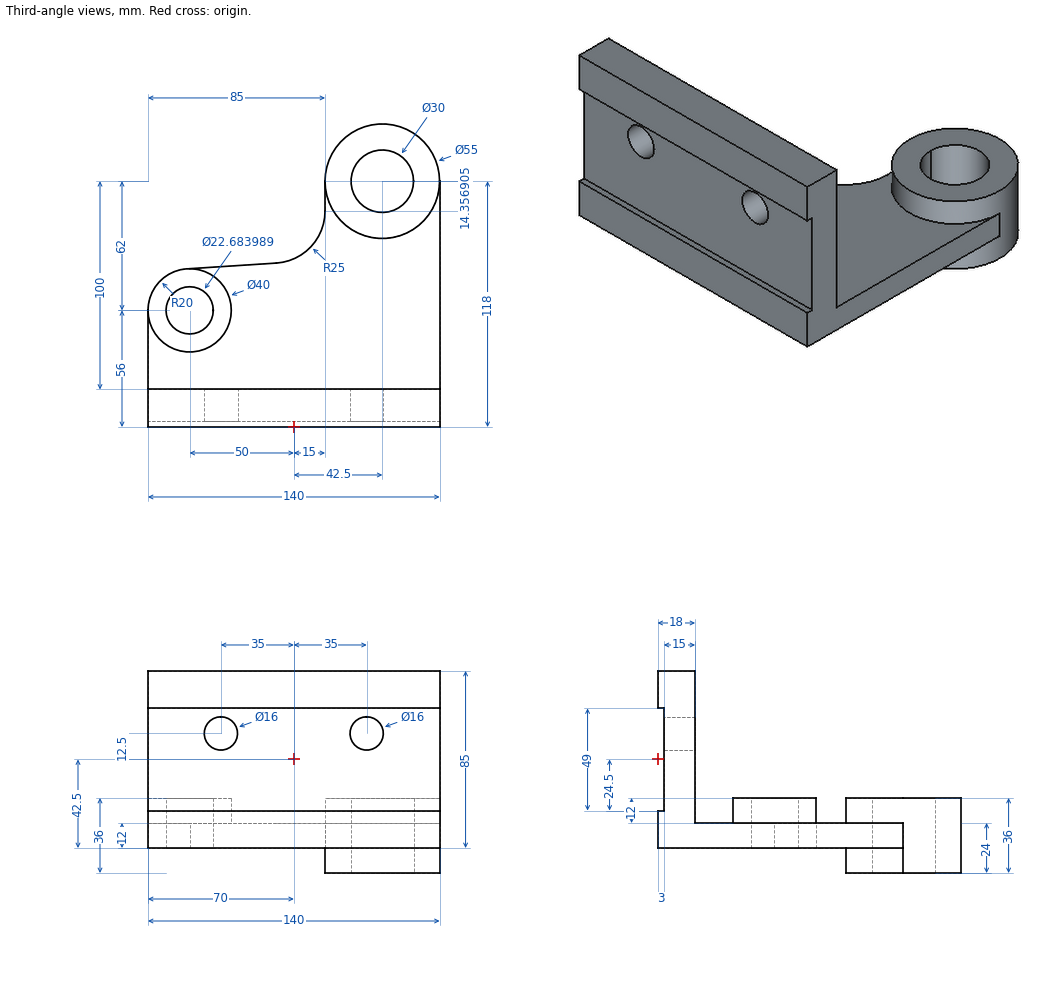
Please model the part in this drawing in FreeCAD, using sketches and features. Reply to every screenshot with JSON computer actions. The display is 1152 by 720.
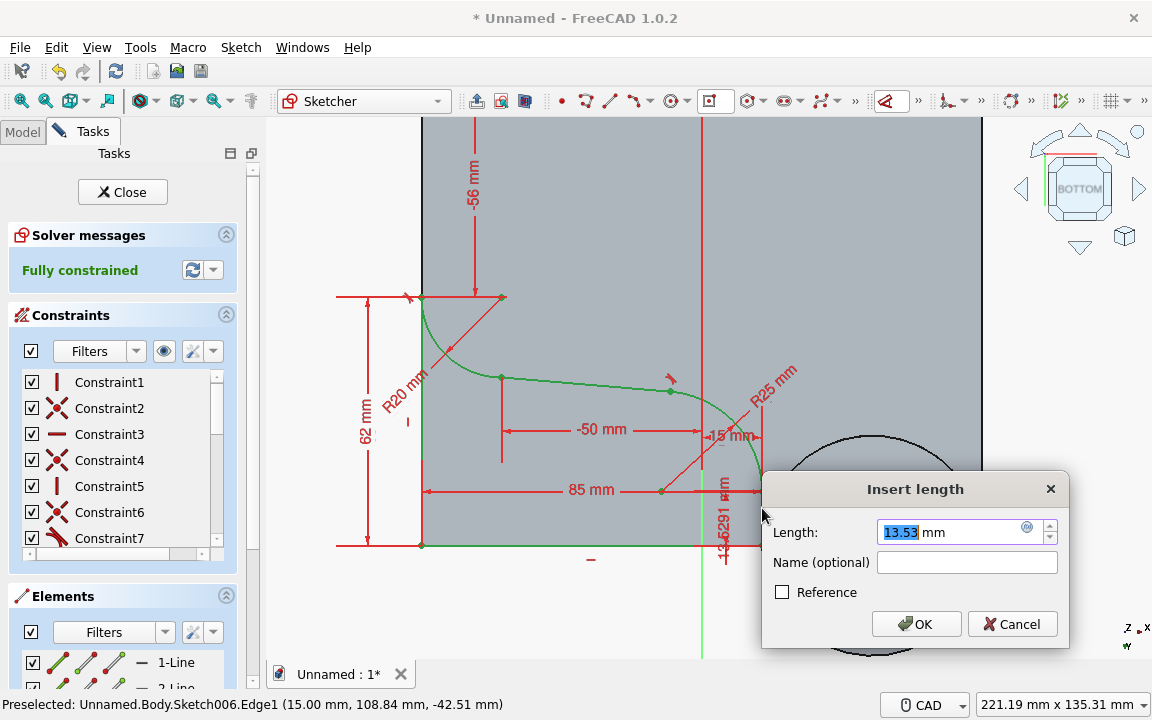
{"action": "type", "text": "14.356905"}
{"action": "key", "text": "Return"}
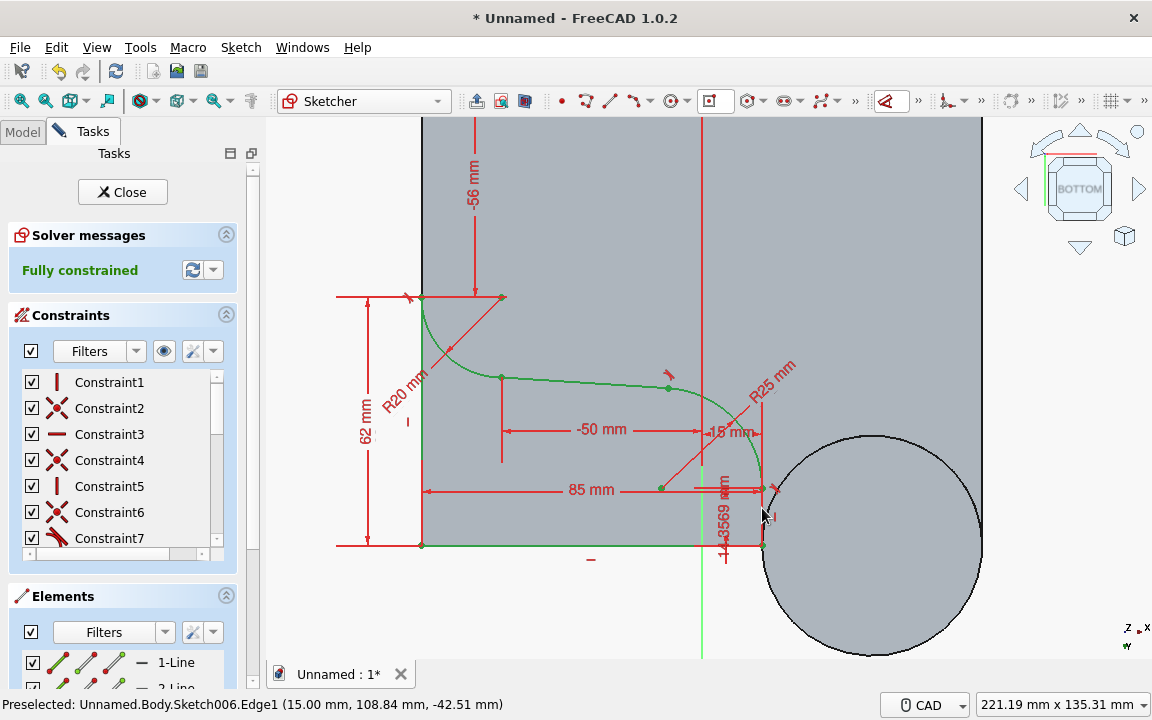
{"action": "left_click", "coordinate": [123, 192]}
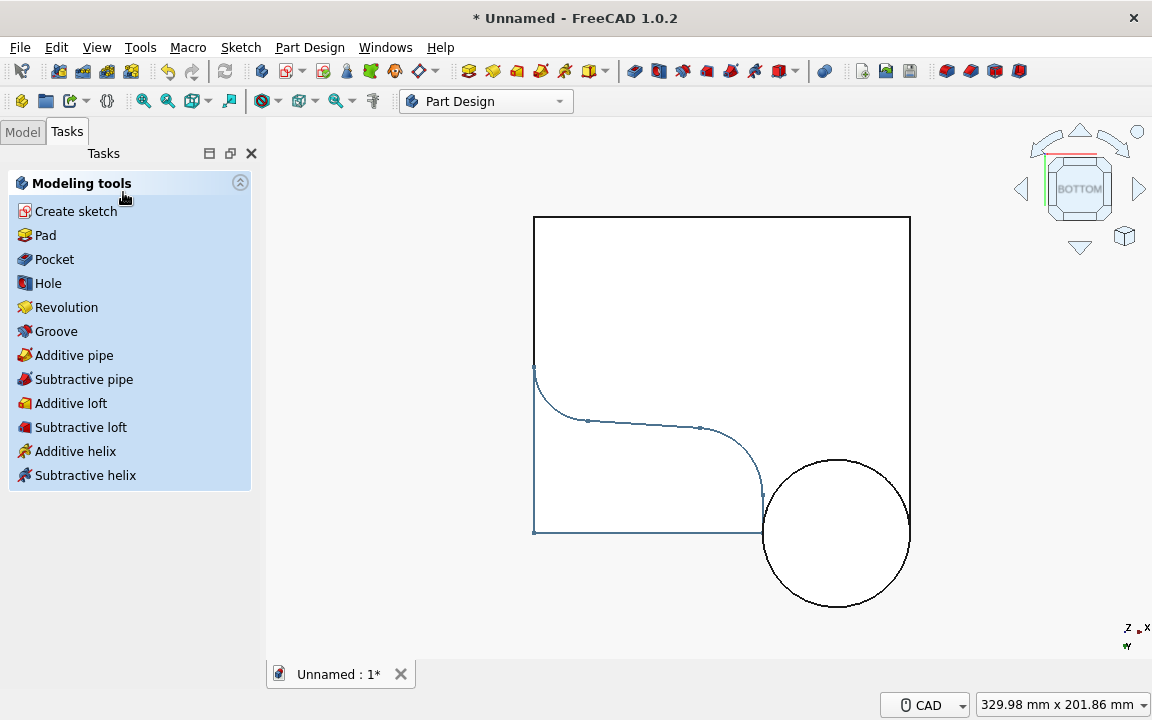
{"action": "left_click", "coordinate": [636, 72]}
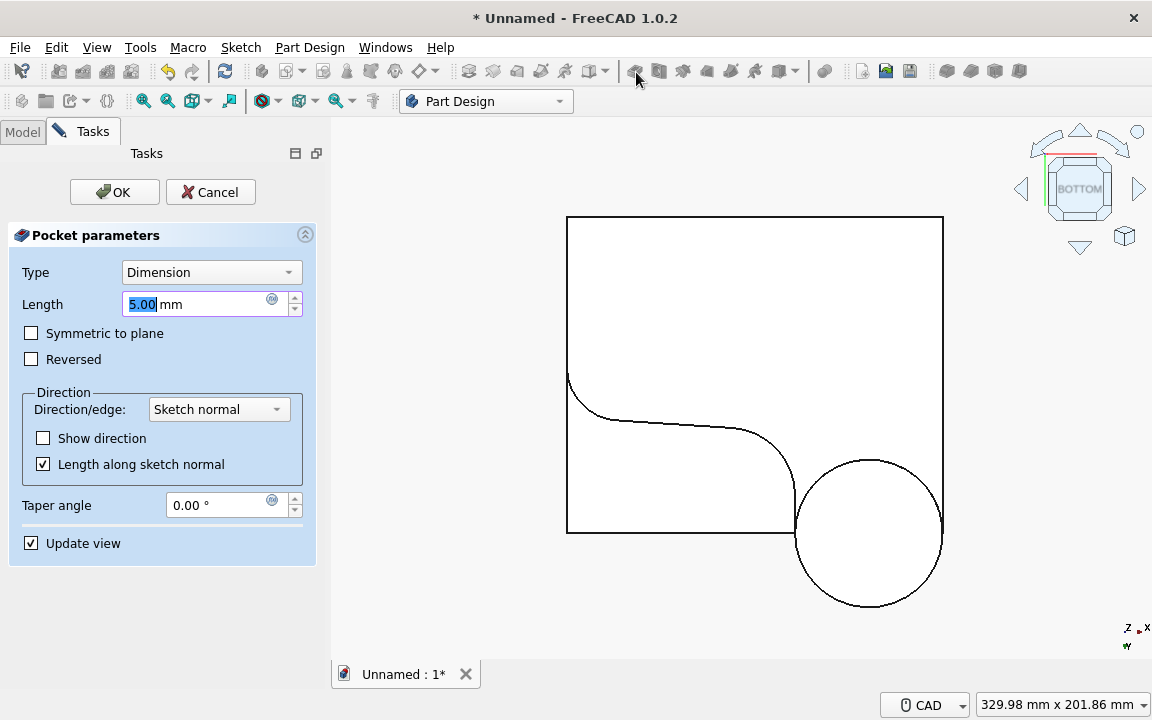
{"action": "type", "text": "12"}
{"action": "key", "text": "Tab"}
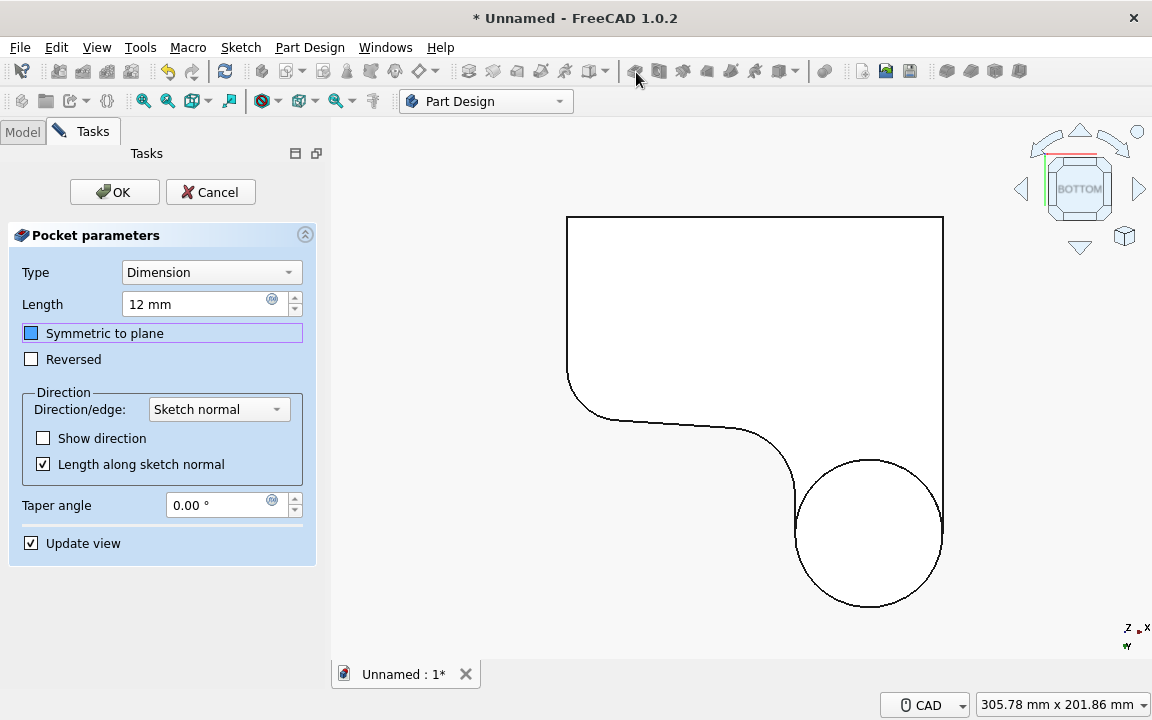
{"action": "left_click", "coordinate": [115, 192]}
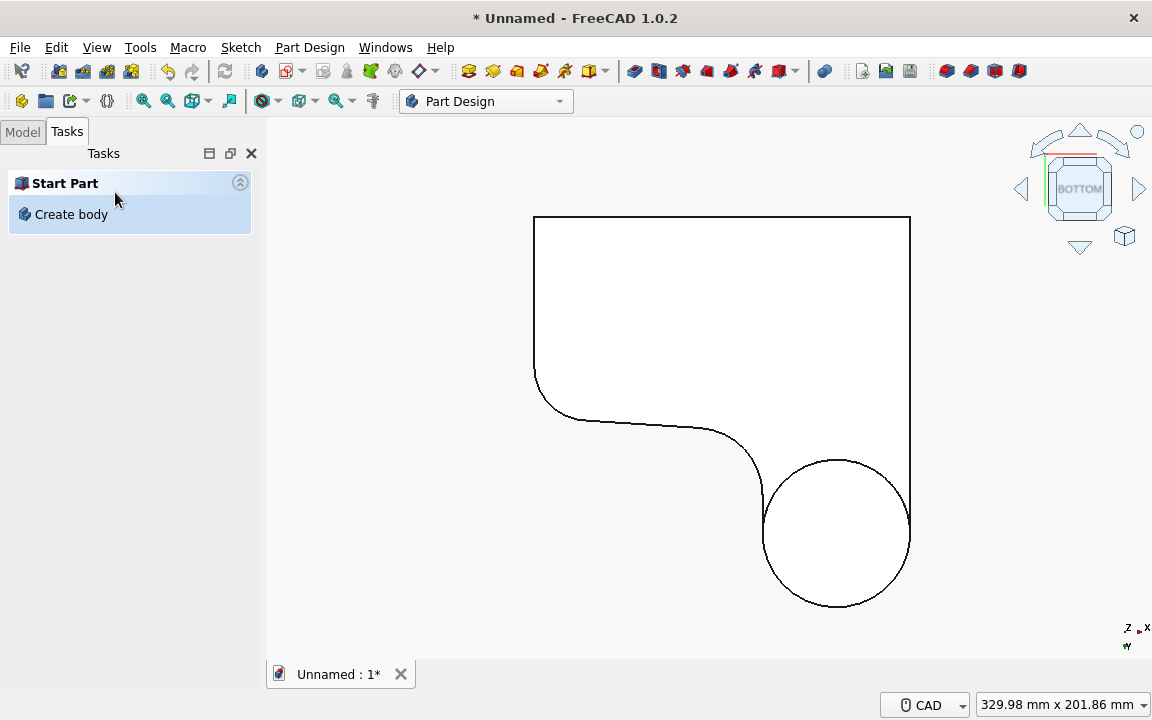
{"action": "key", "text": "0"}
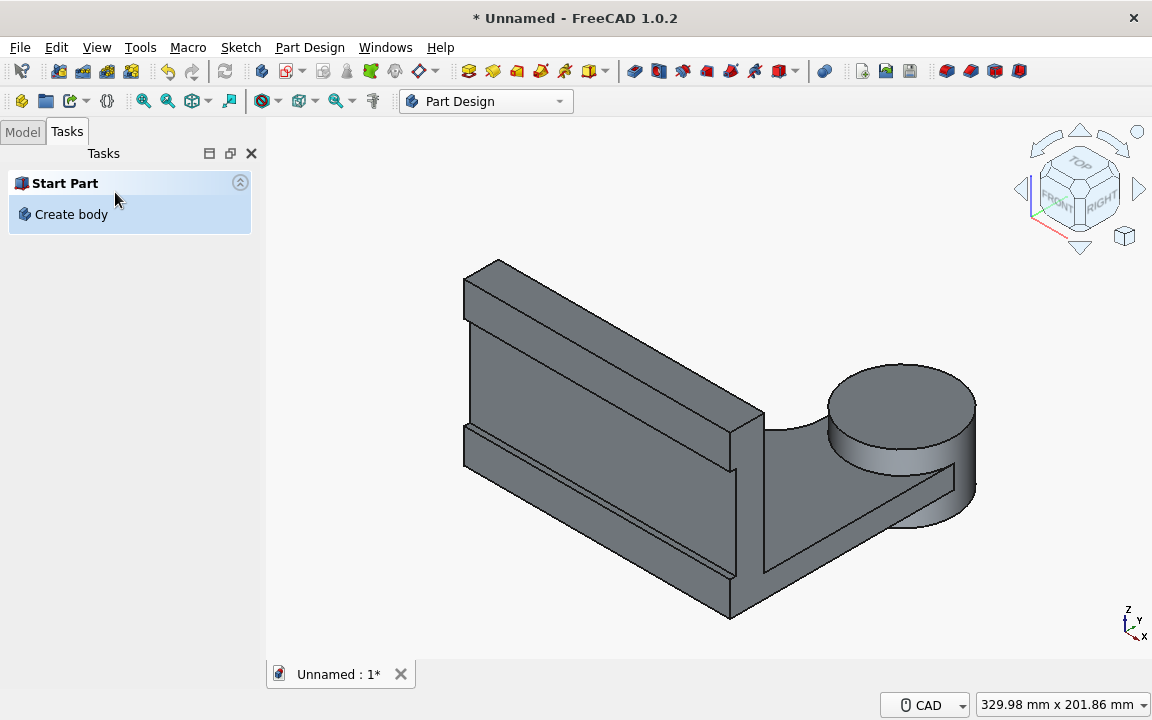
{"action": "left_click", "coordinate": [902, 406]}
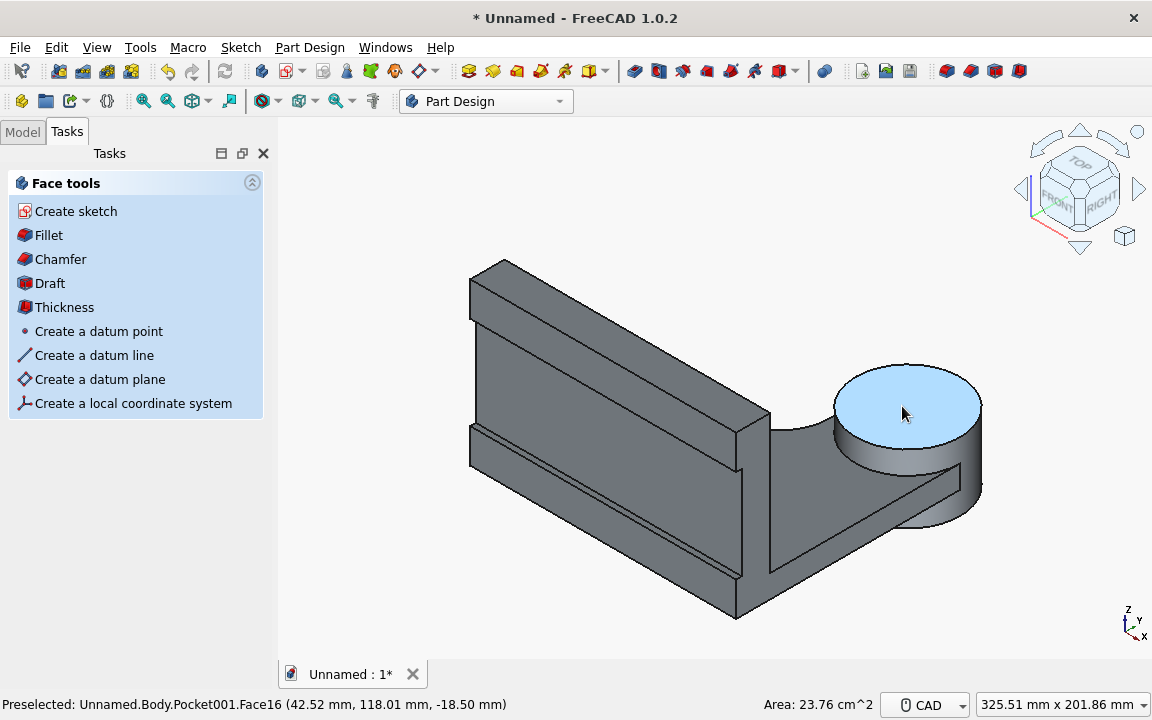
{"action": "left_click", "coordinate": [286, 72]}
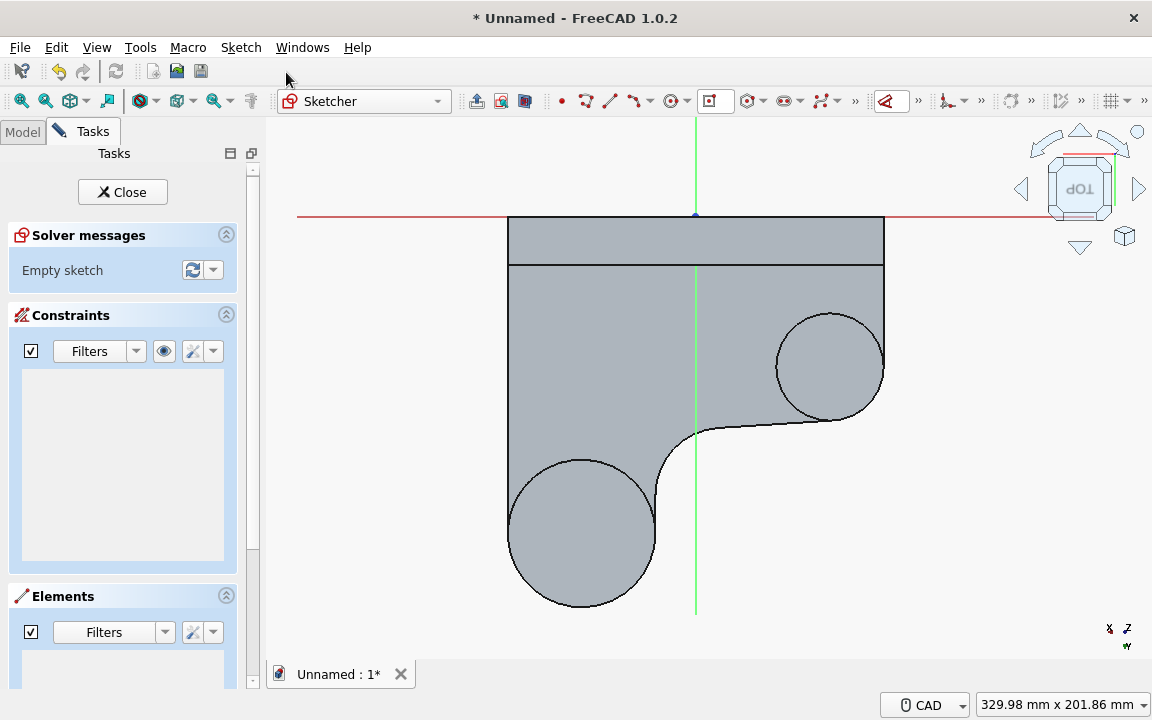
{"action": "scroll", "coordinate": [562, 581], "scroll_direction": "up", "scroll_amount": 7}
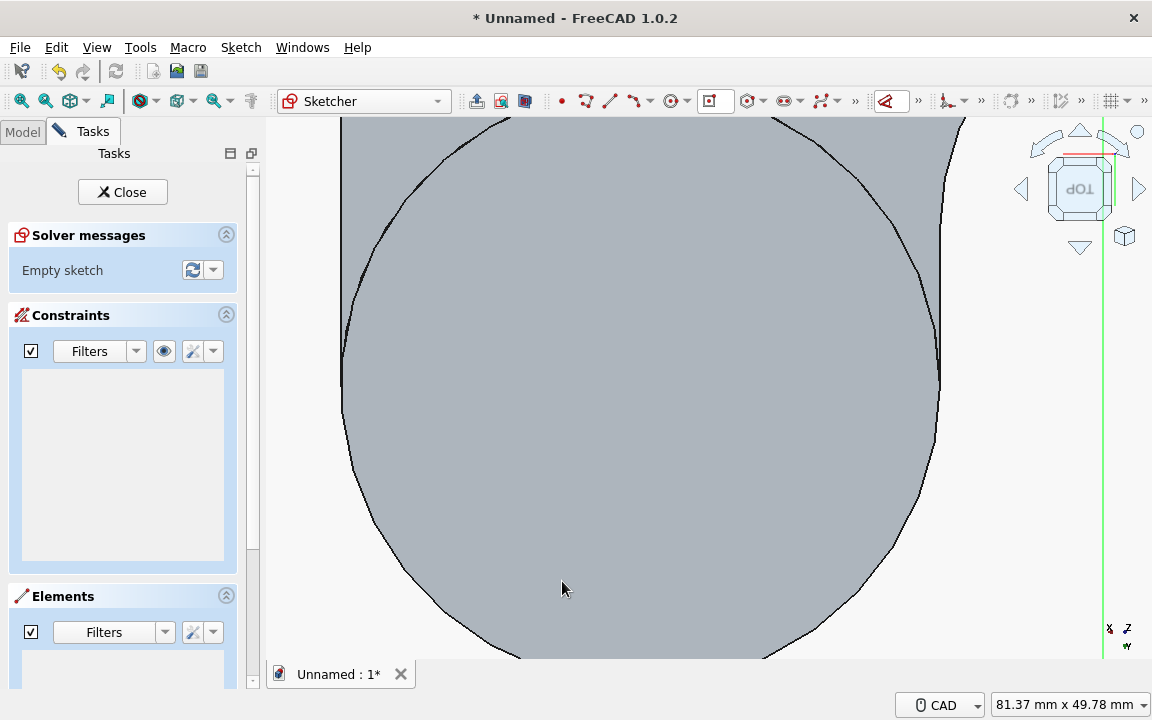
{"action": "left_click", "coordinate": [672, 102]}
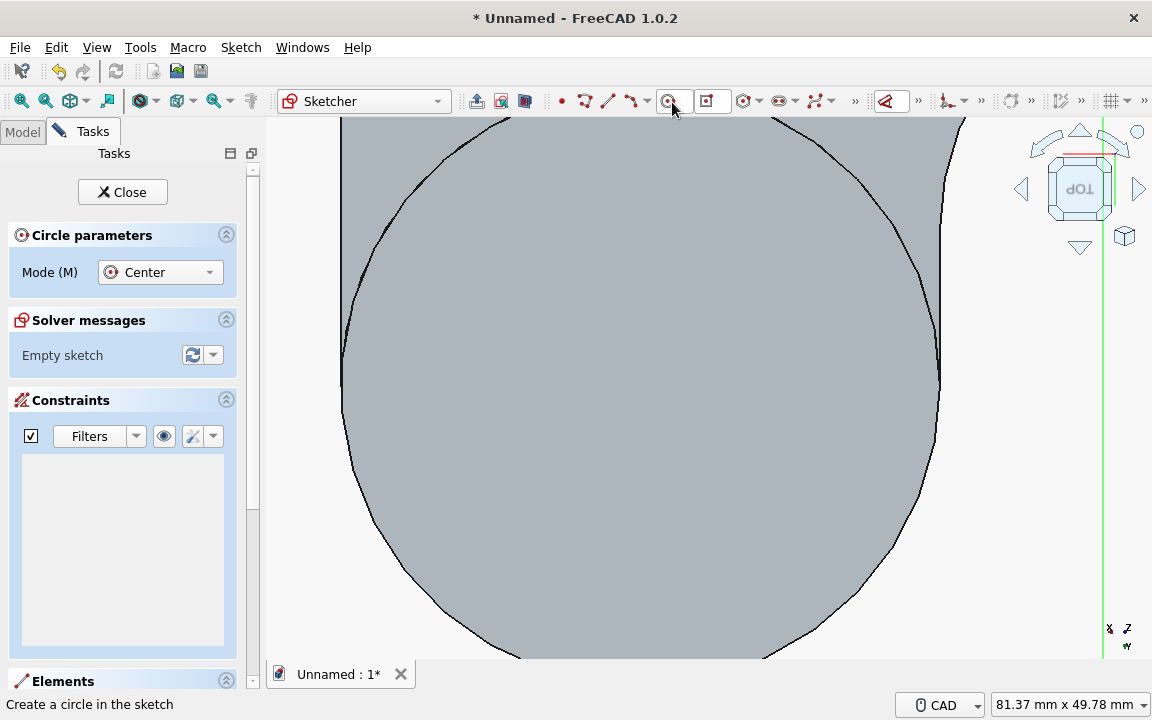
{"action": "left_click", "coordinate": [641, 386]}
{"action": "left_click", "coordinate": [756, 270]}
{"action": "key", "text": "Escape"}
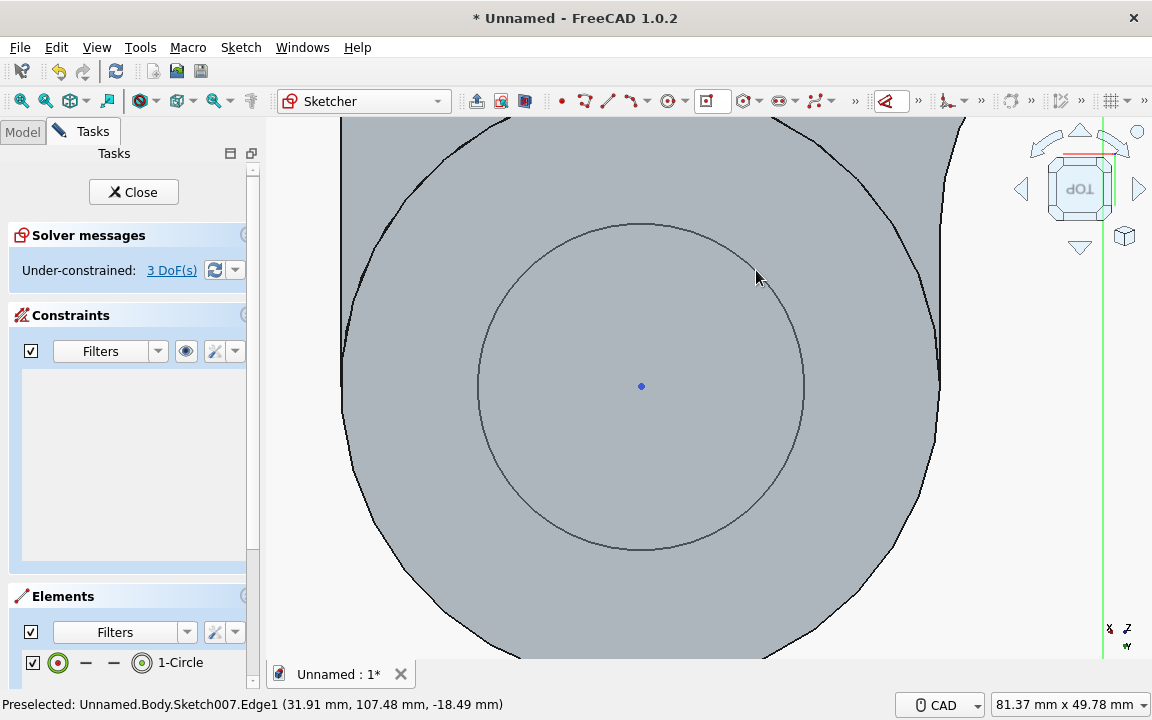
{"action": "left_click", "coordinate": [756, 271]}